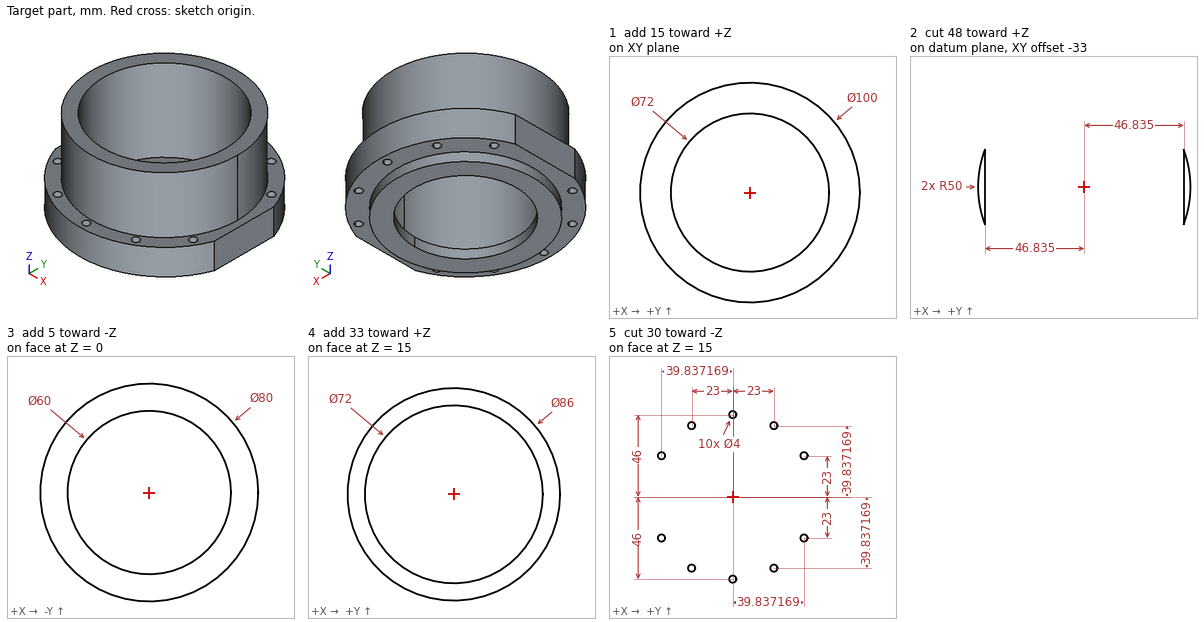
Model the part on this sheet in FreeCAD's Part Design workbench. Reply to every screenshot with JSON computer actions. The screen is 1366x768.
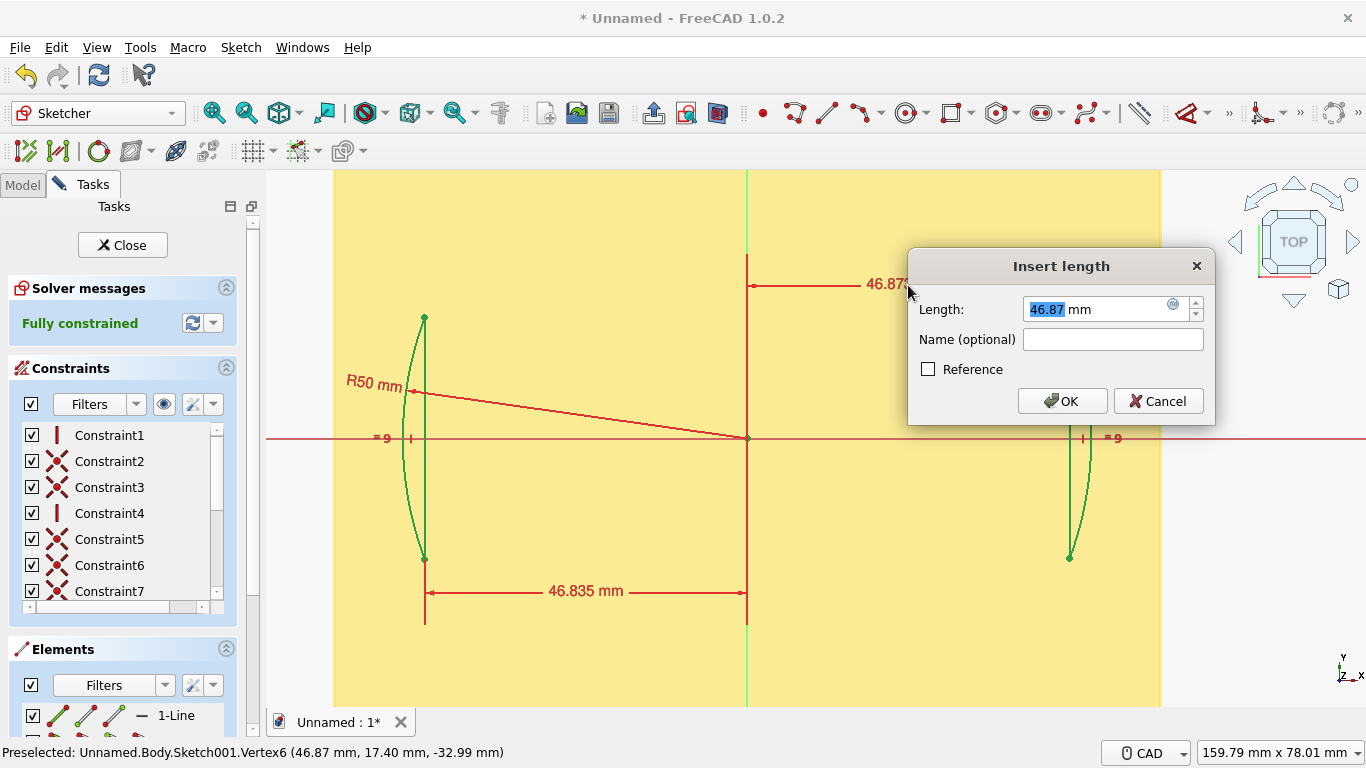
{"action": "type", "text": "46.835"}
{"action": "key", "text": "Return"}
{"action": "key", "text": "Escape"}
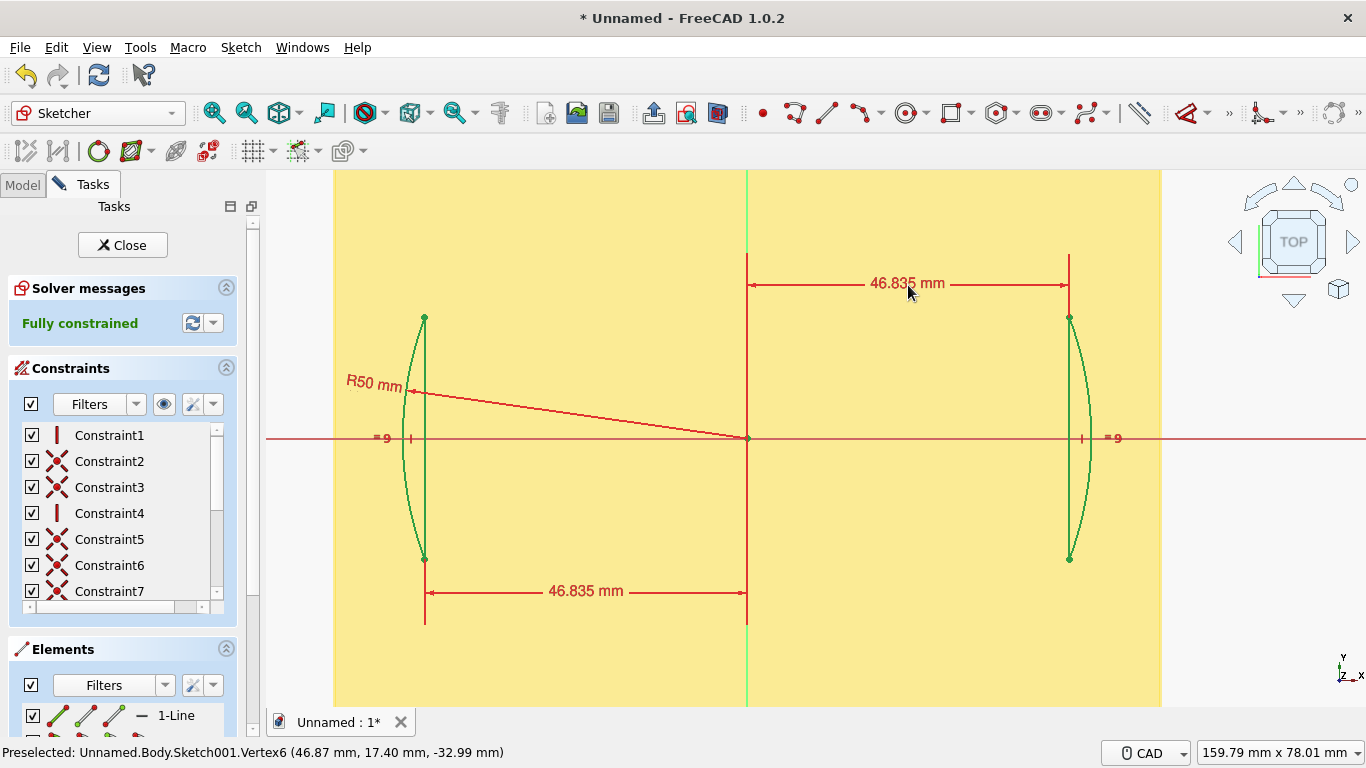
{"action": "left_click", "coordinate": [123, 245]}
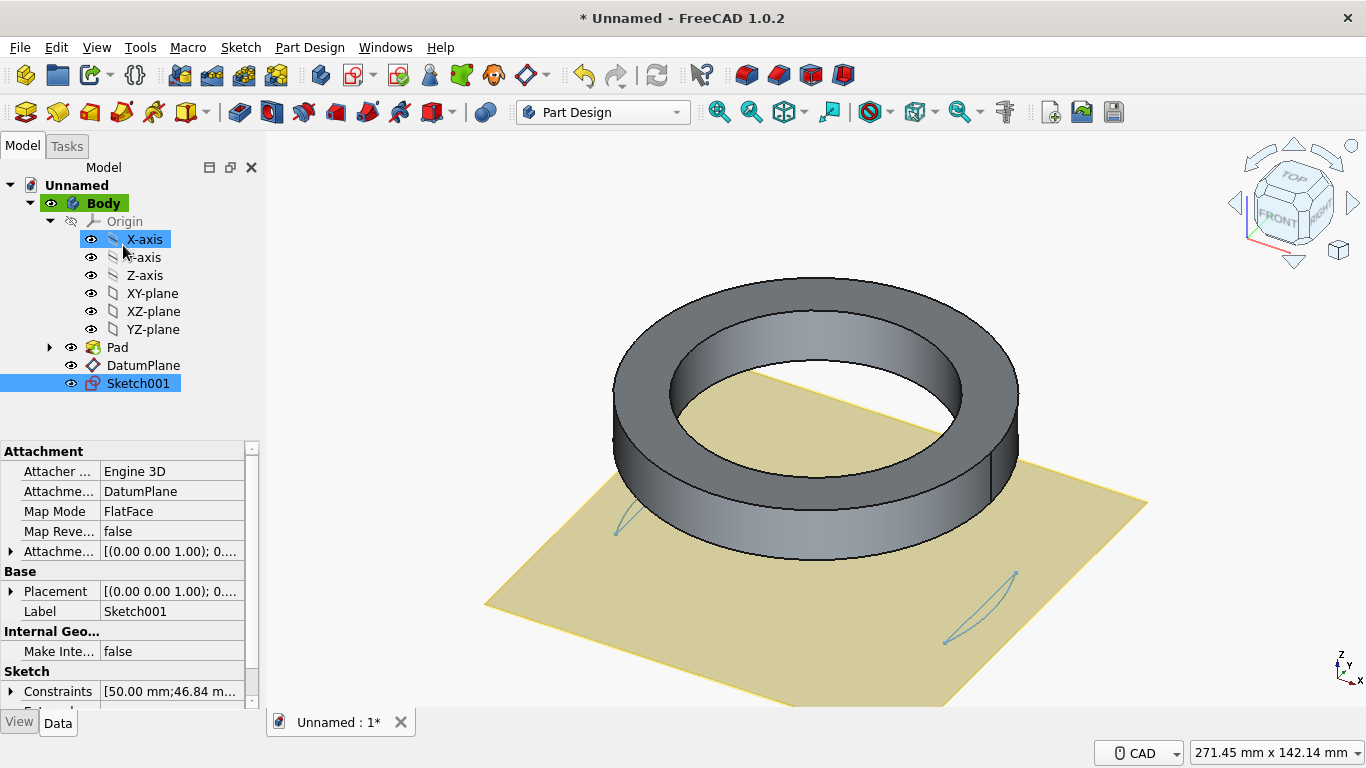
{"action": "left_click", "coordinate": [240, 112]}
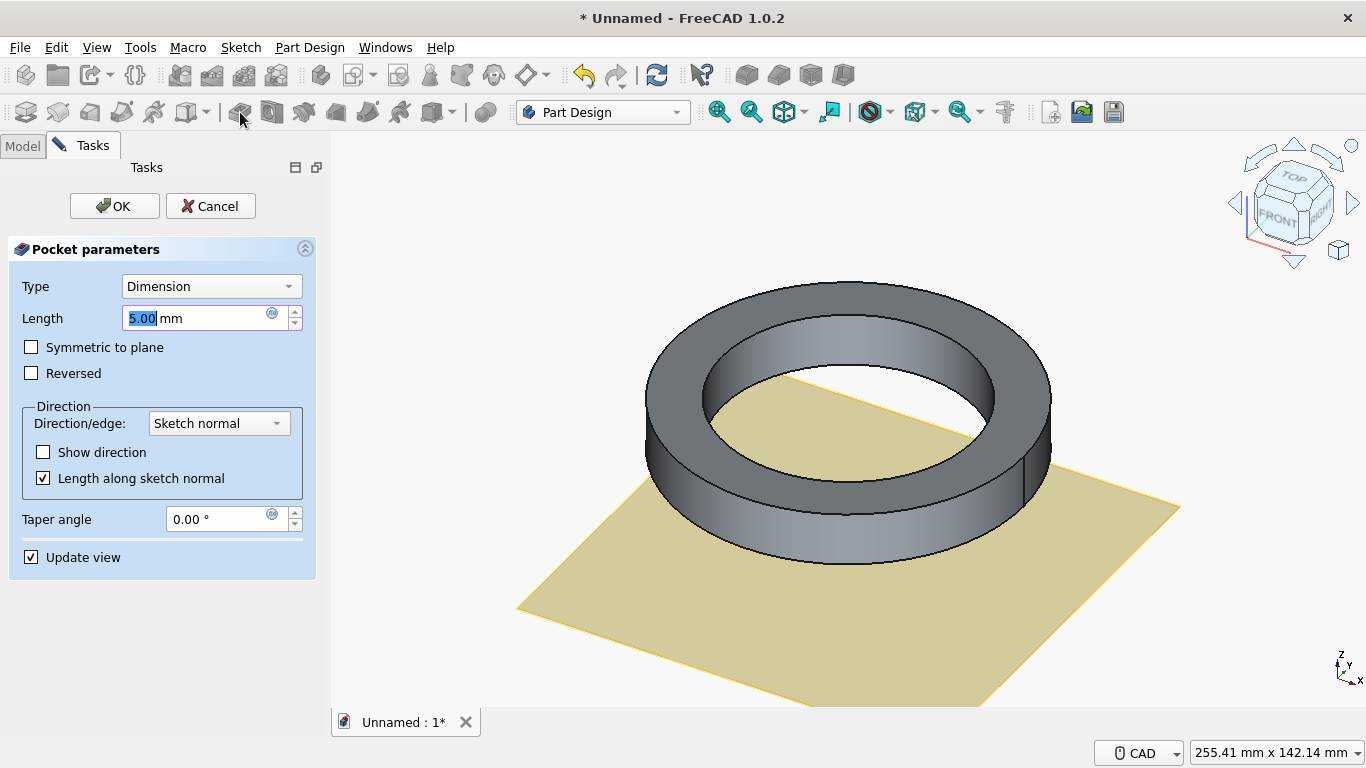
{"action": "type", "text": "48"}
{"action": "key", "text": "Tab"}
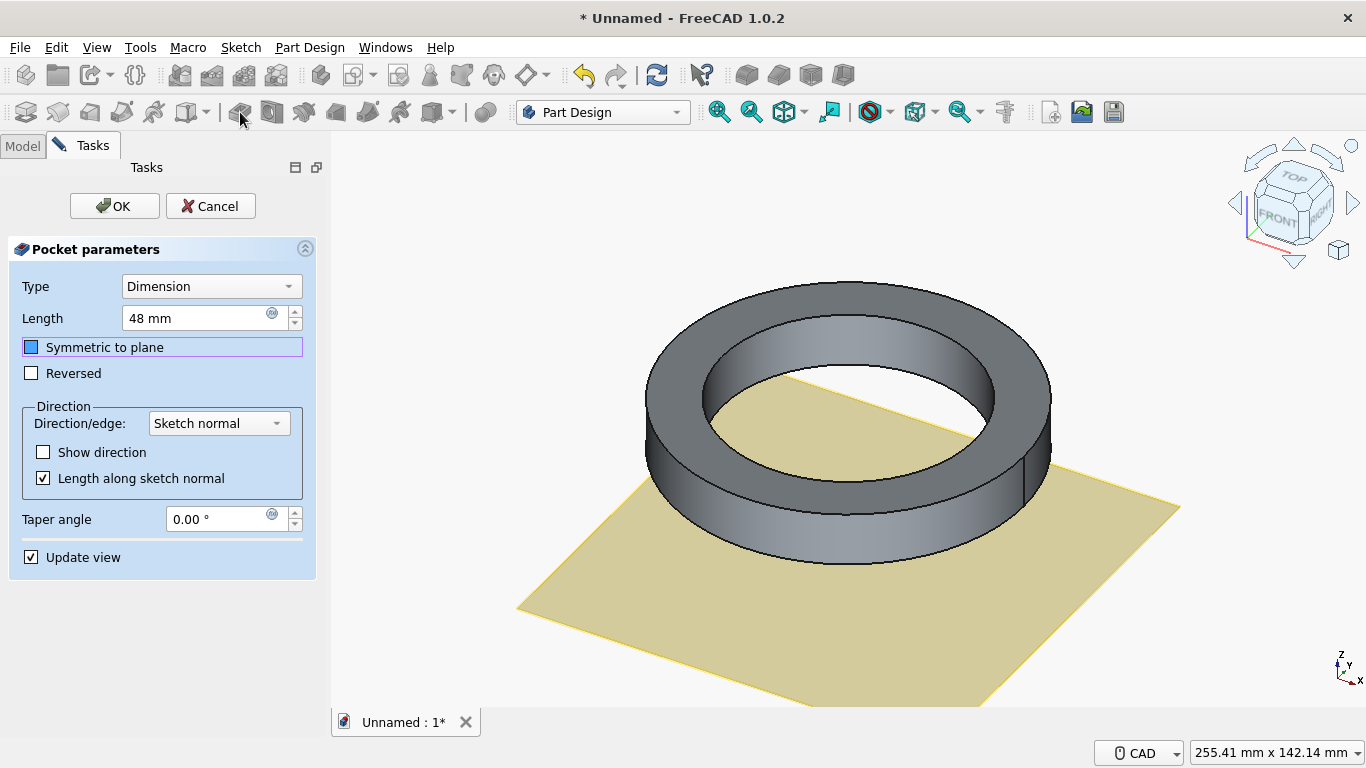
{"action": "left_click", "coordinate": [30, 373]}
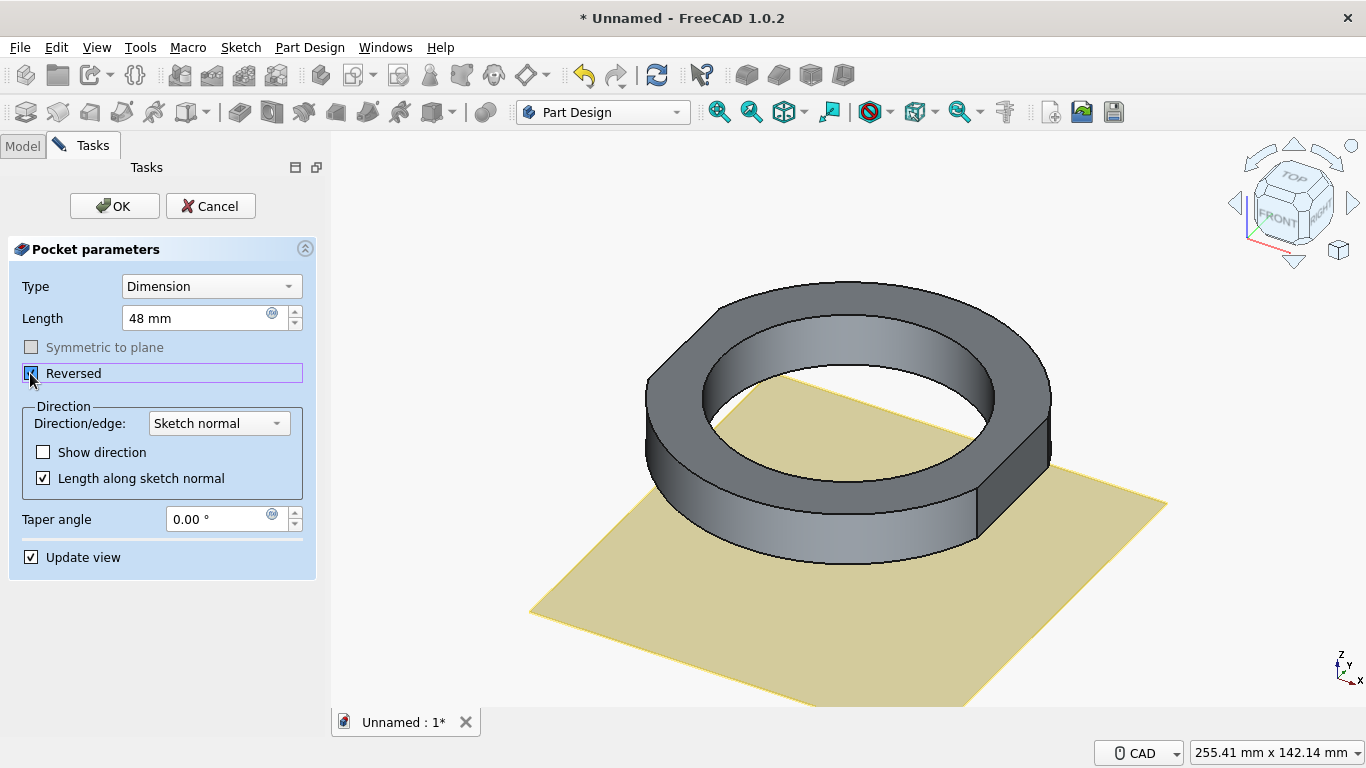
{"action": "left_click", "coordinate": [115, 206]}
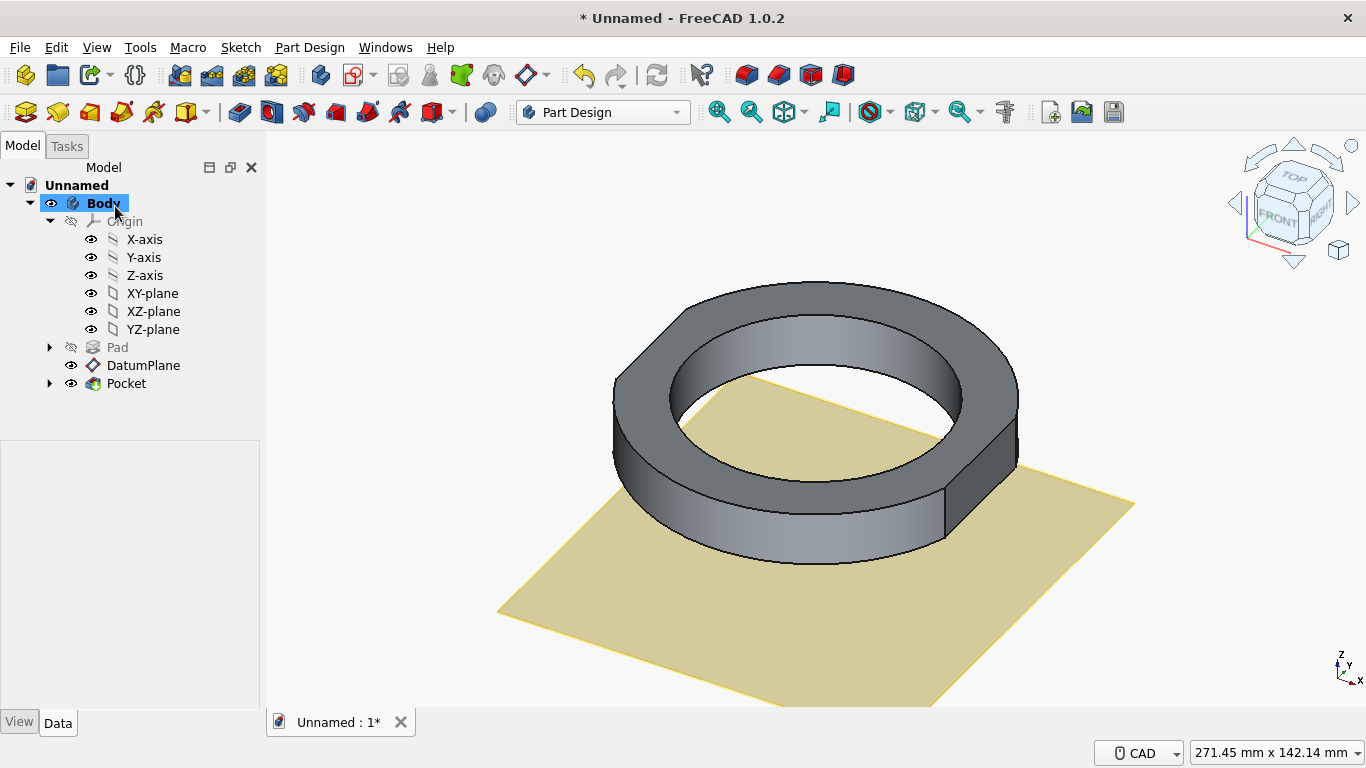
{"action": "left_click", "coordinate": [116, 365]}
{"action": "key", "text": "space"}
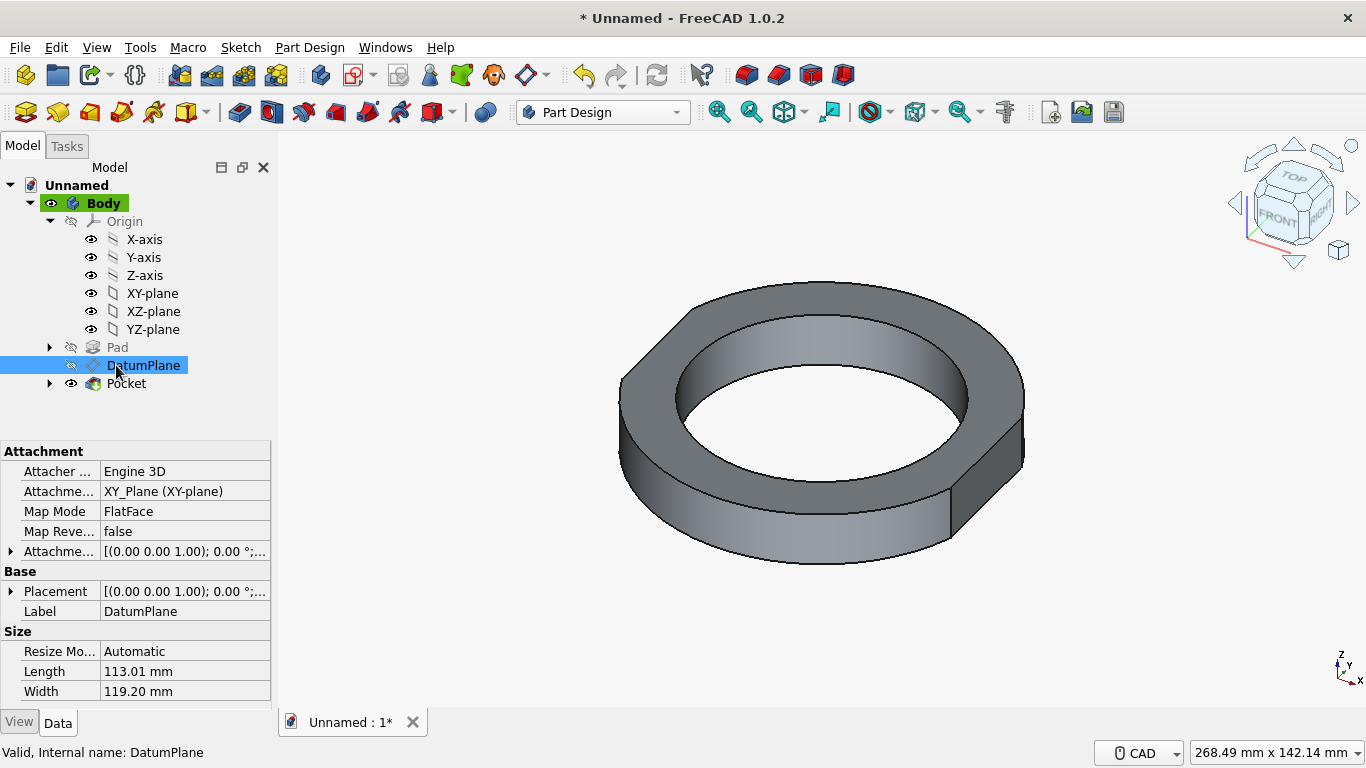
{"action": "key", "text": "5"}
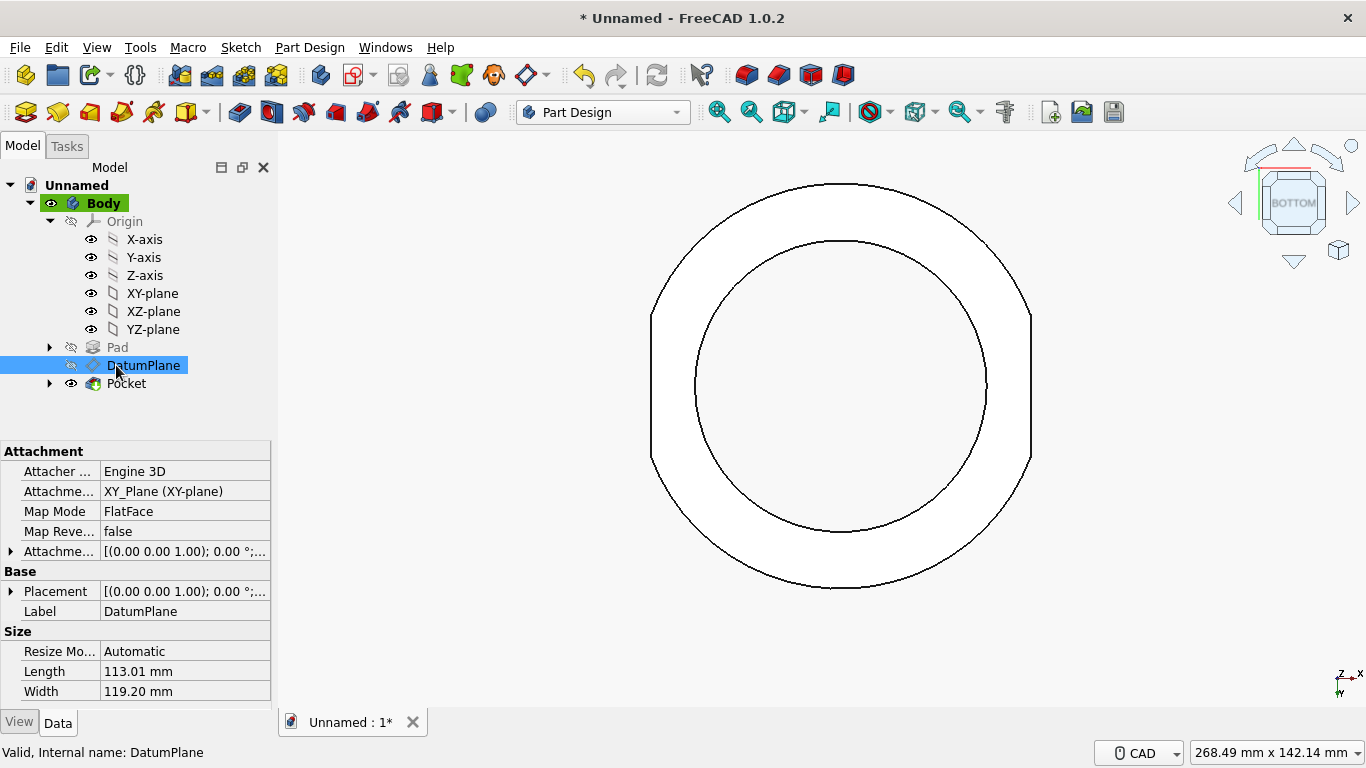
{"action": "left_click", "coordinate": [841, 559]}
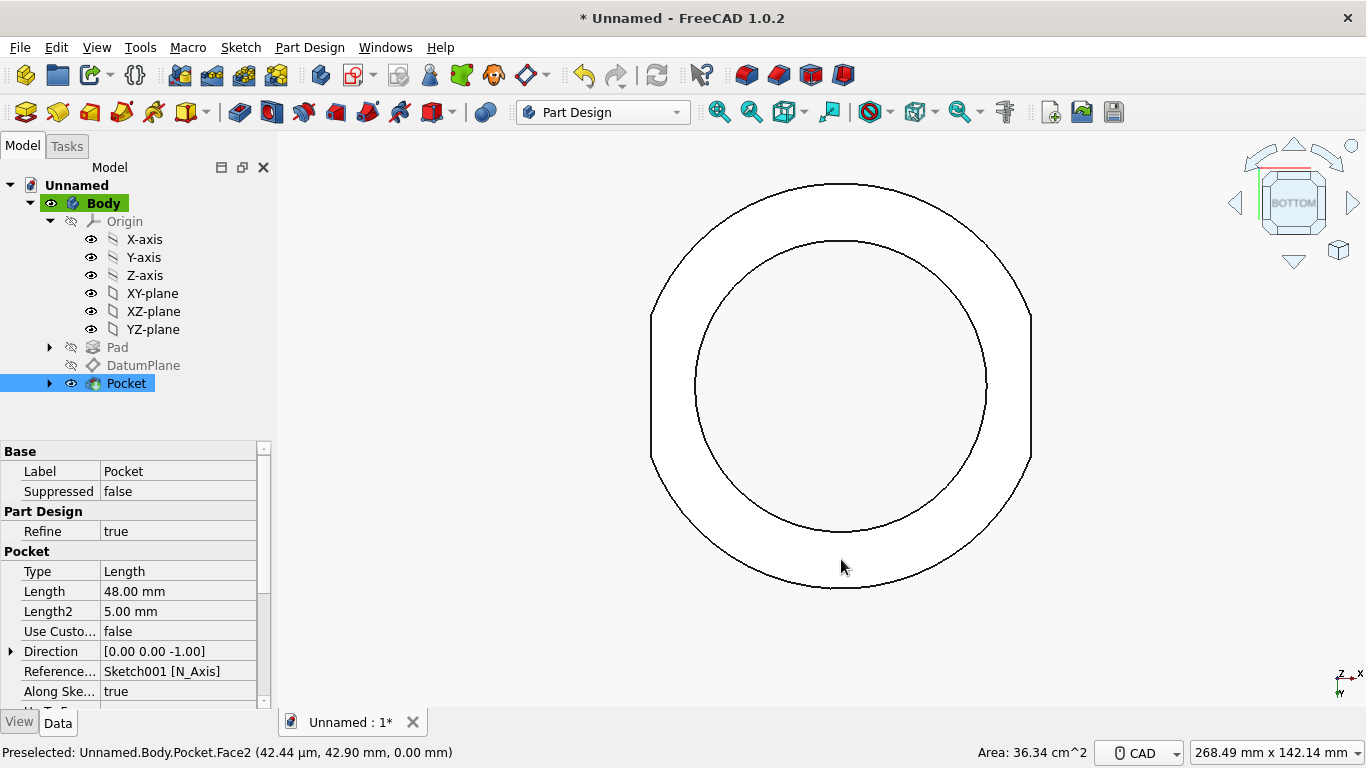
{"action": "left_click", "coordinate": [354, 76]}